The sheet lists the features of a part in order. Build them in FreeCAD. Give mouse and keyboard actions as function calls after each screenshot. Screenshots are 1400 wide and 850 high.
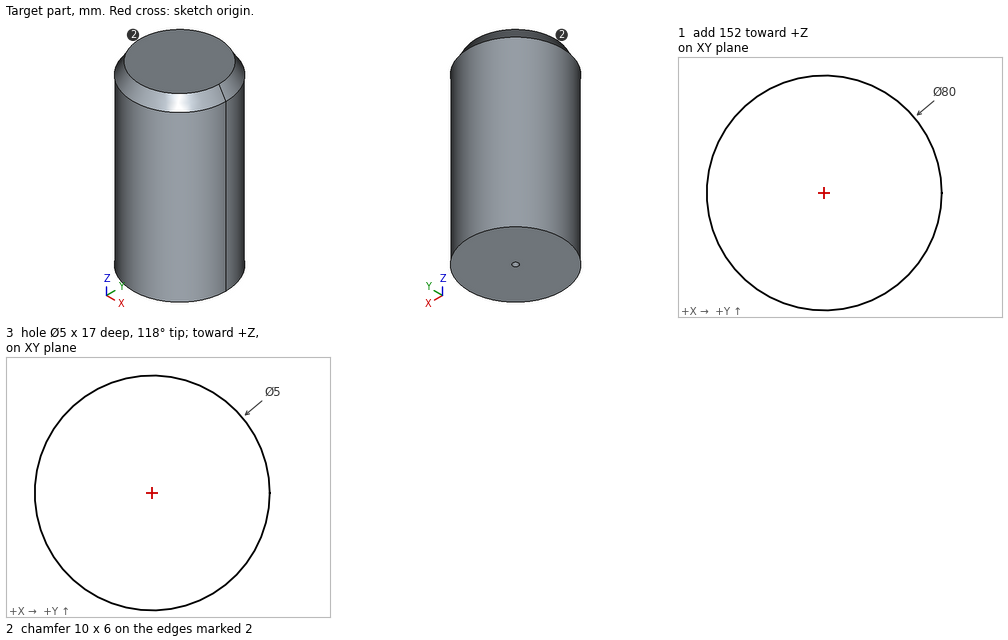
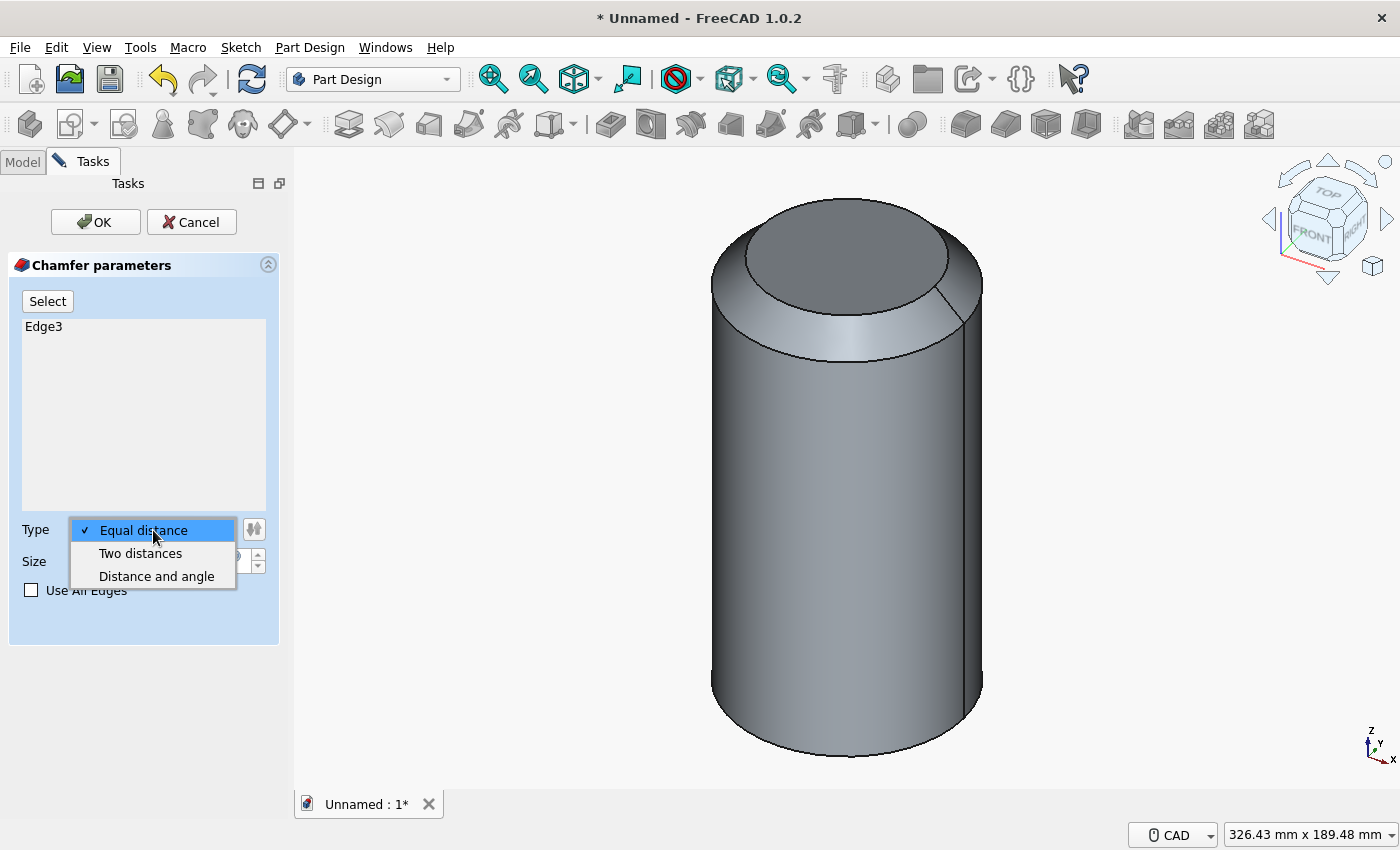
click(152, 554)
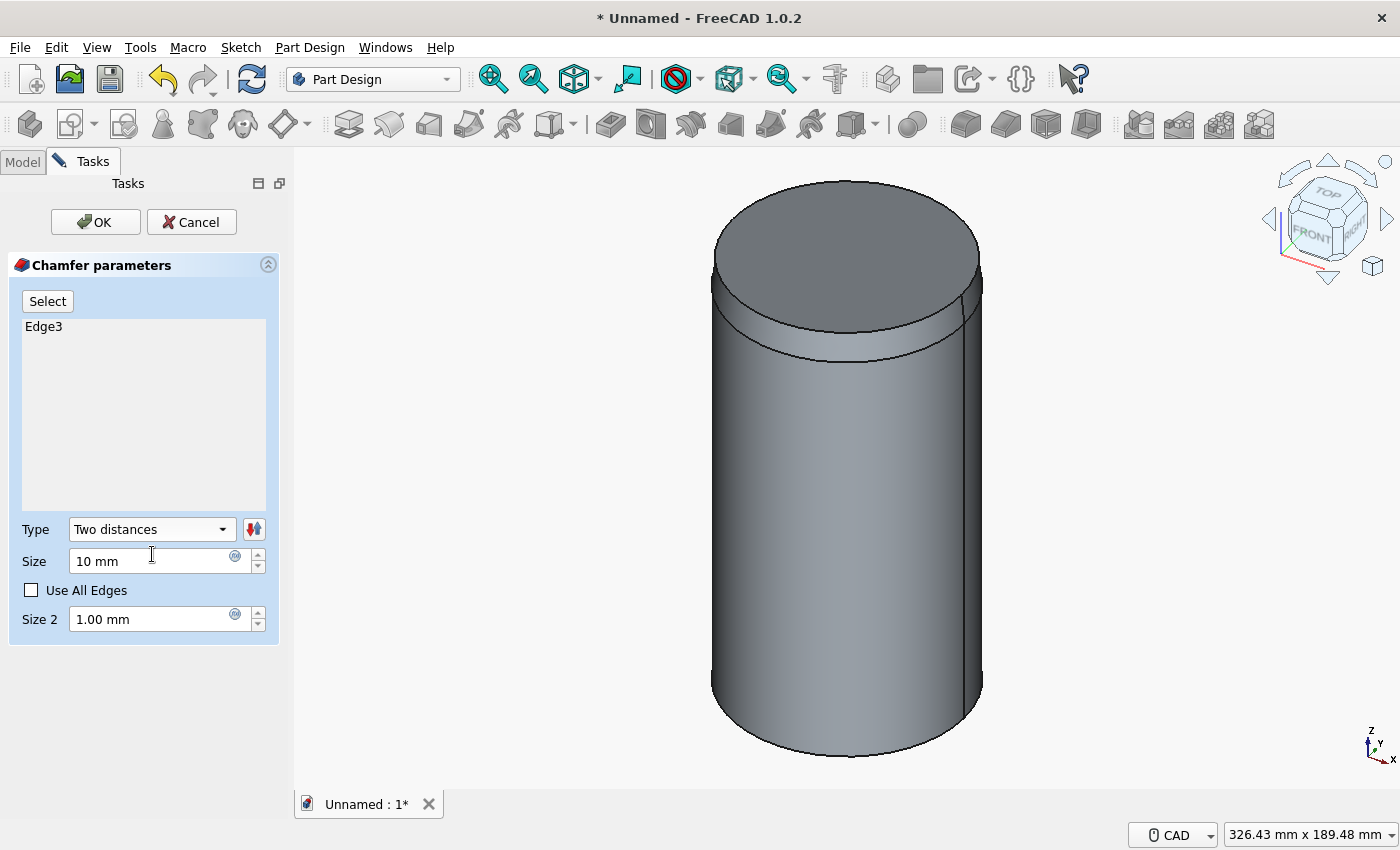
triple_click(160, 619)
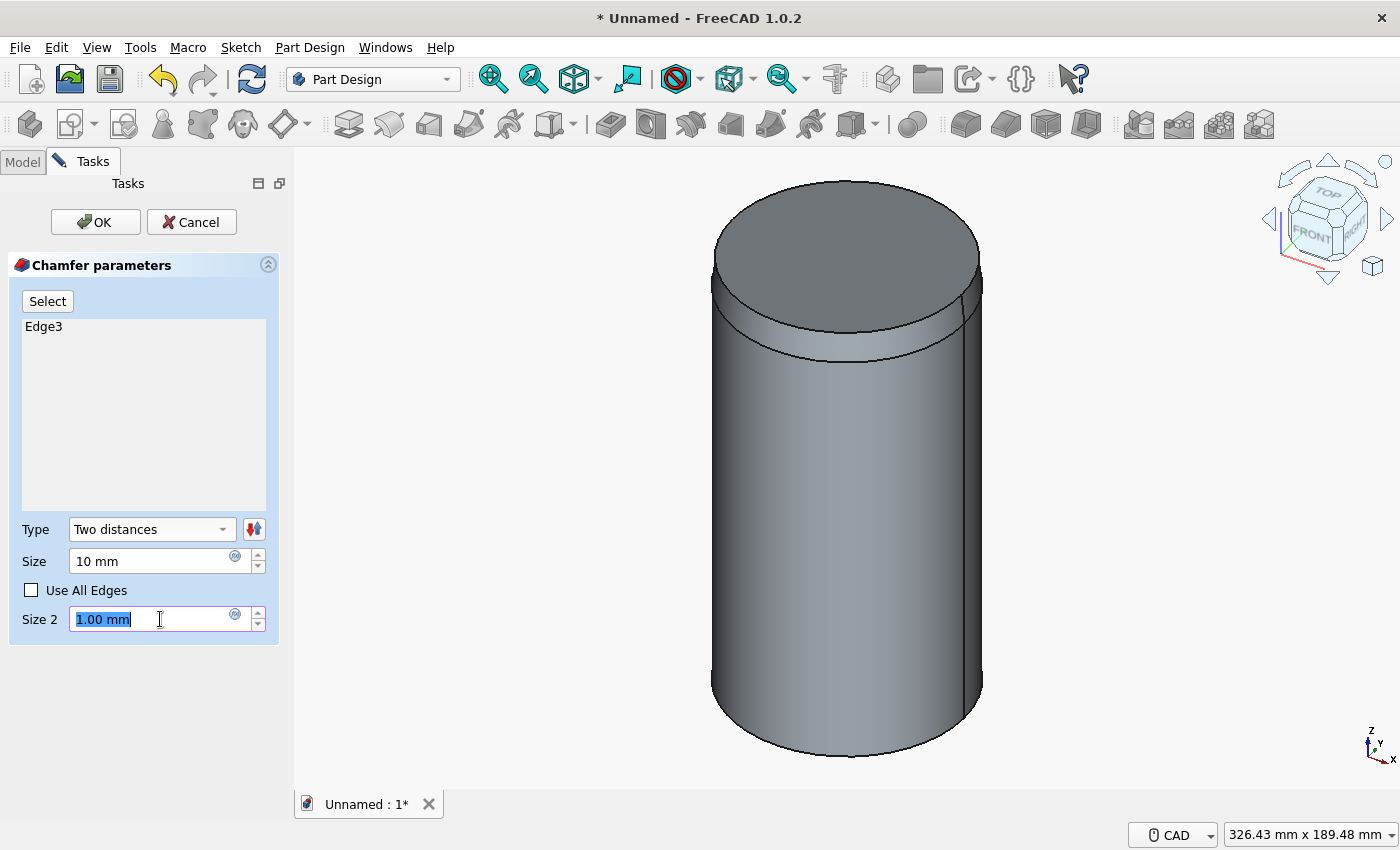
text(6)
key(Tab)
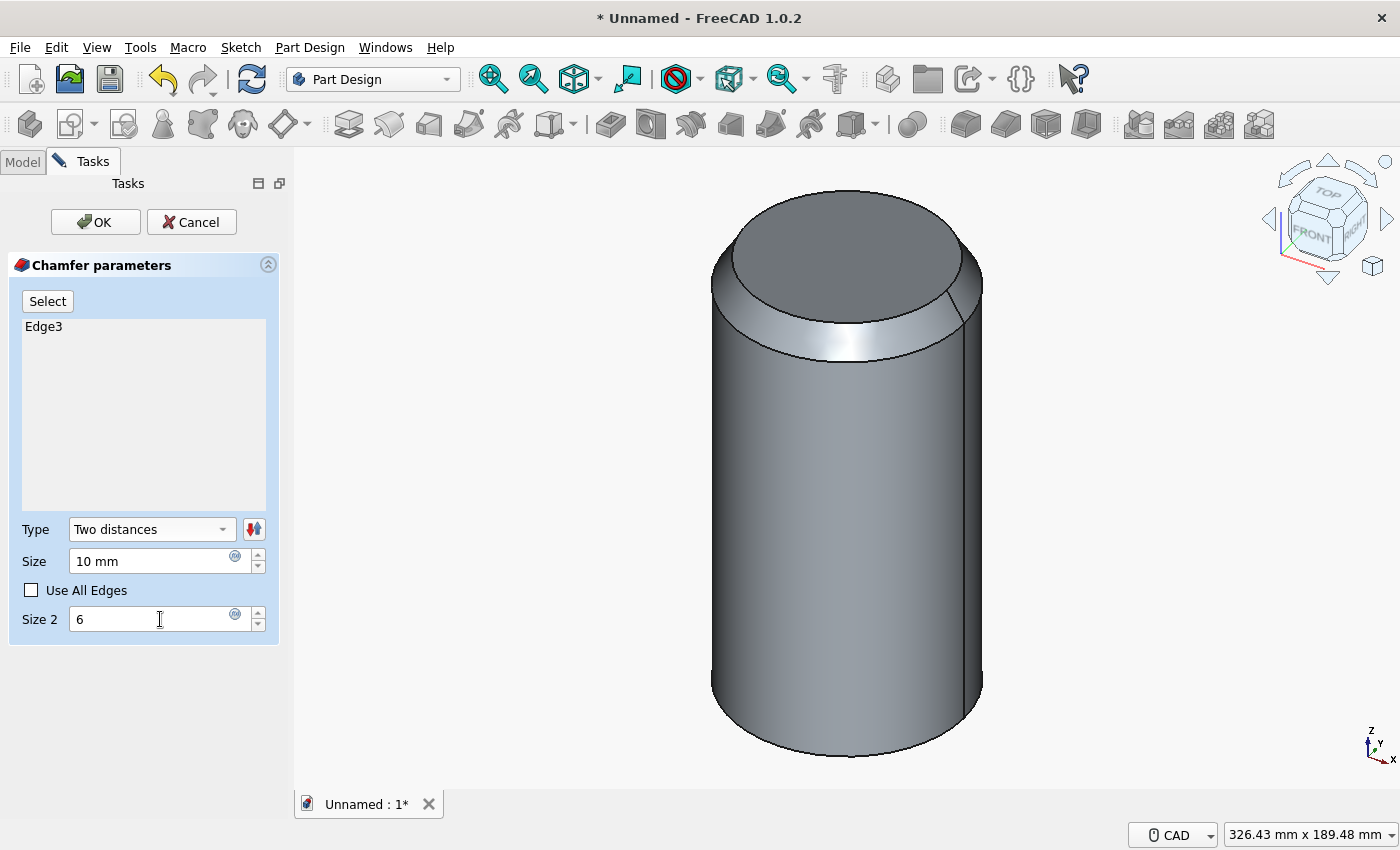
click(96, 222)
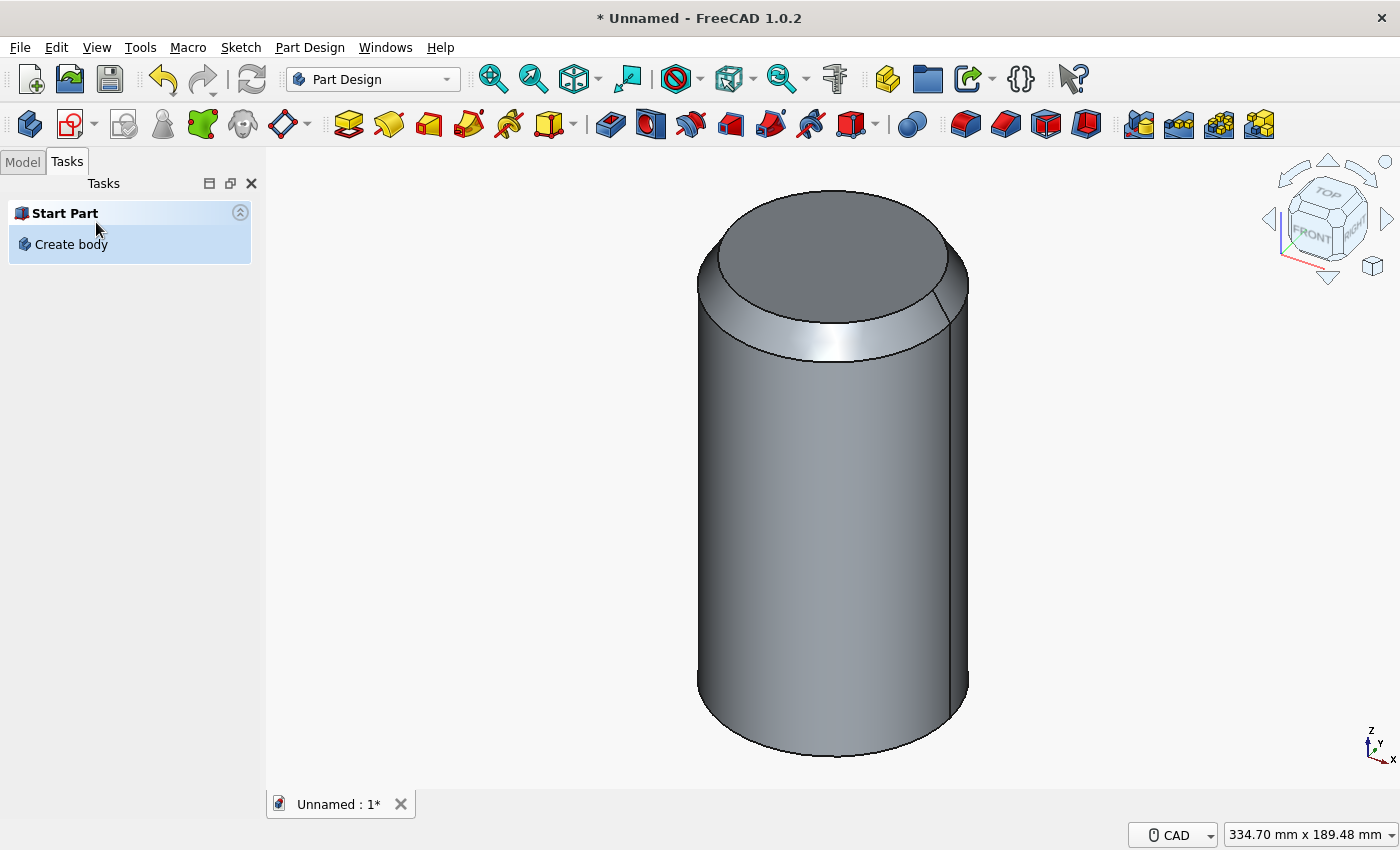
click(70, 124)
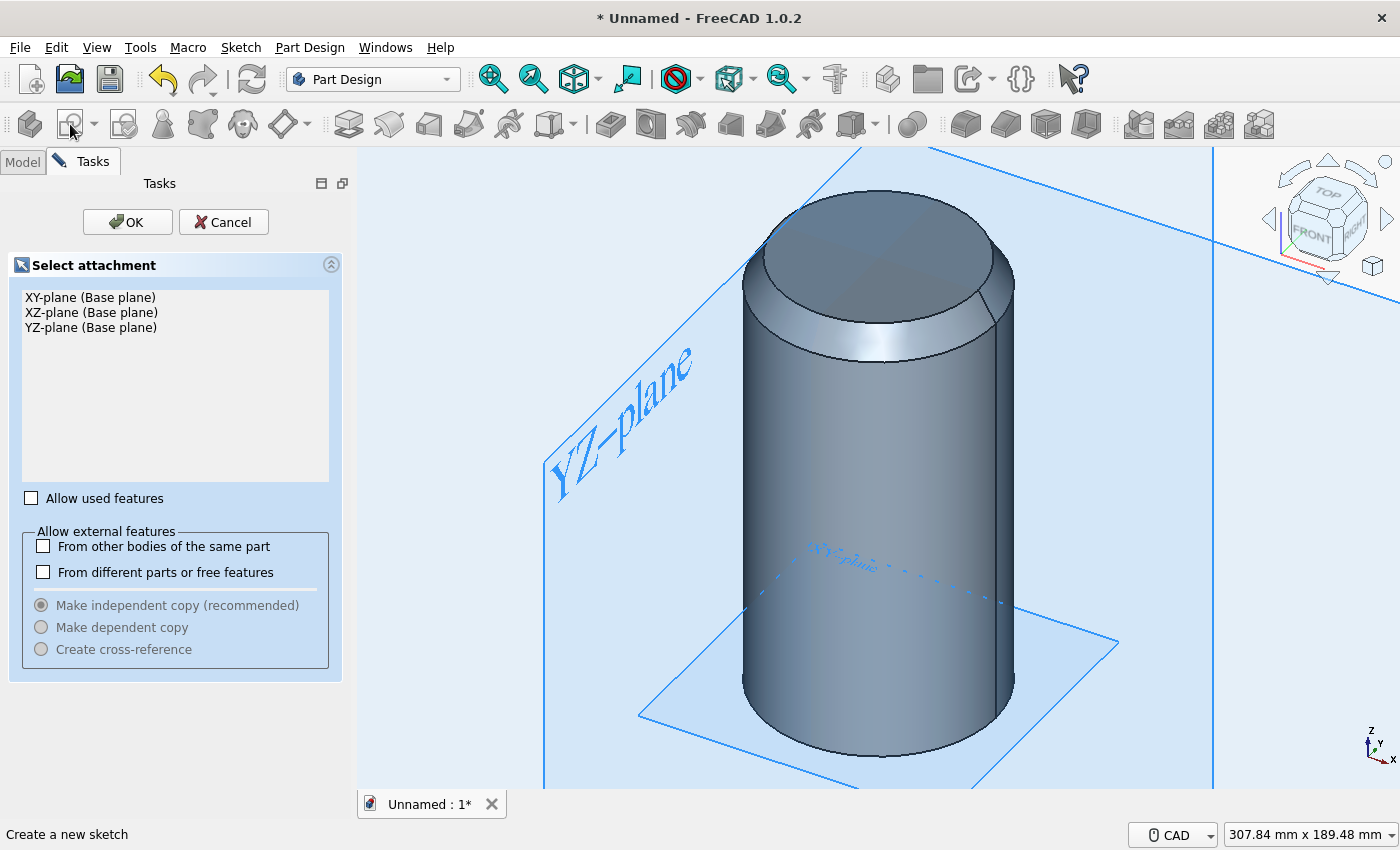
click(82, 298)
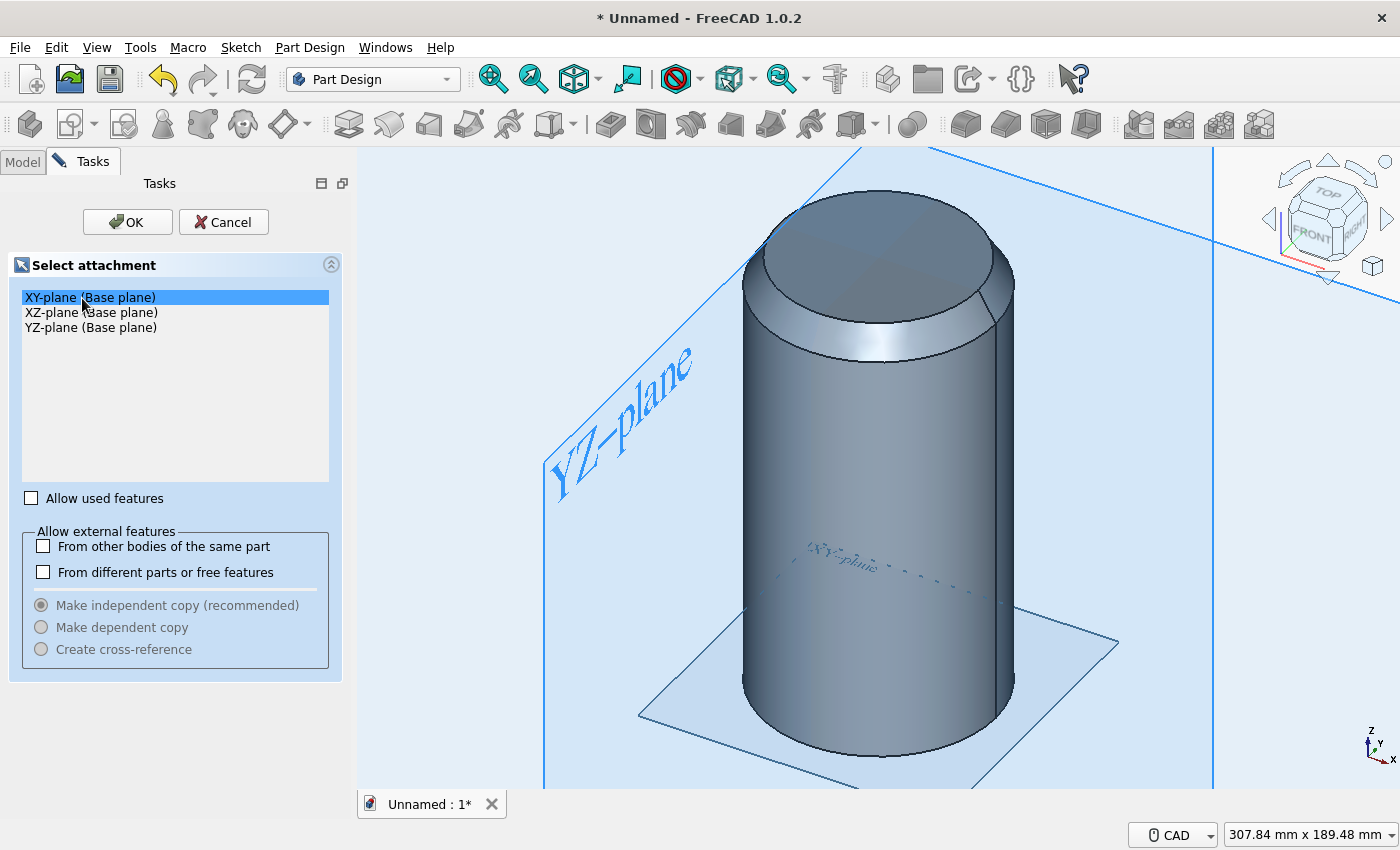
click(128, 222)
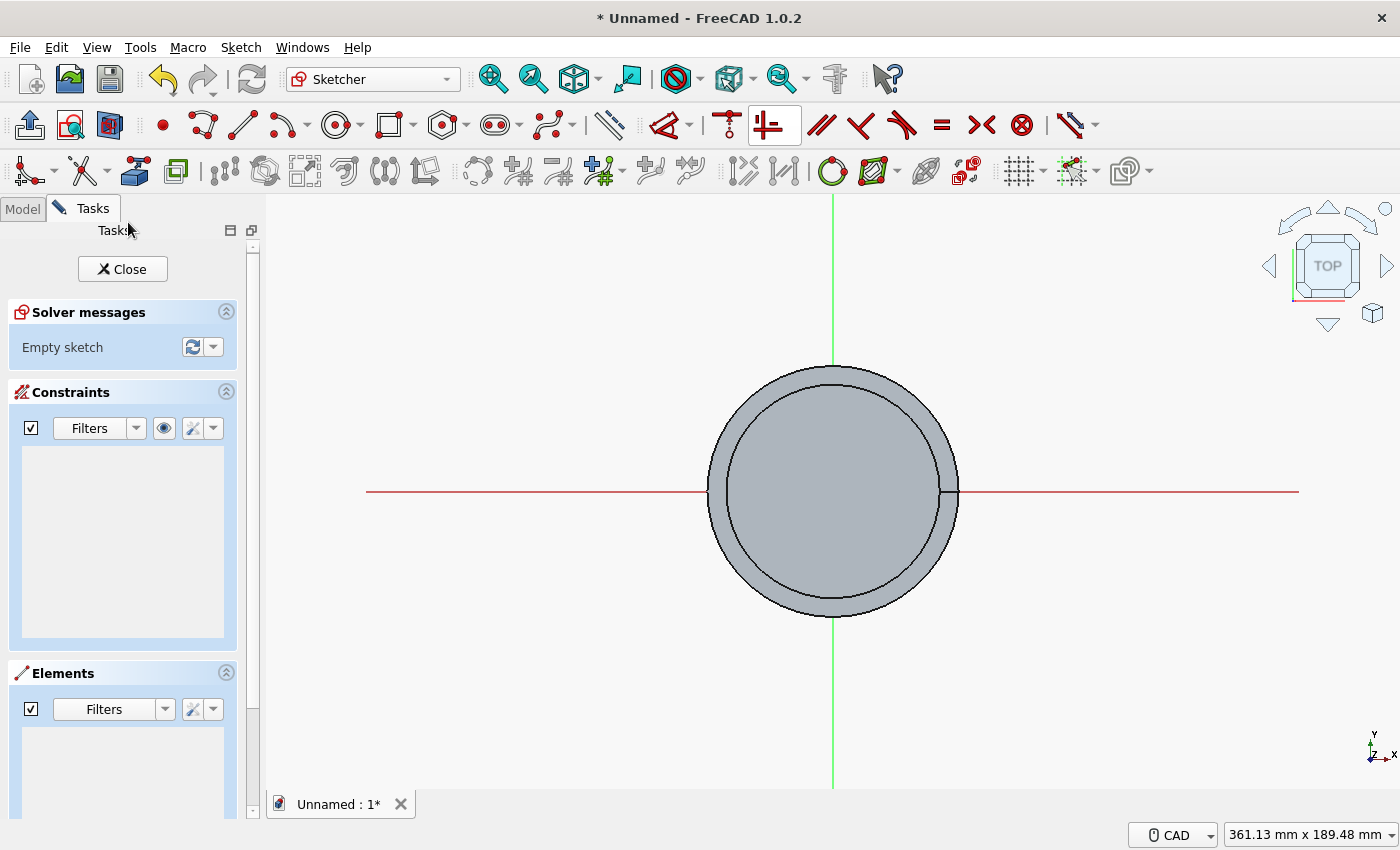
key(q)
key(s)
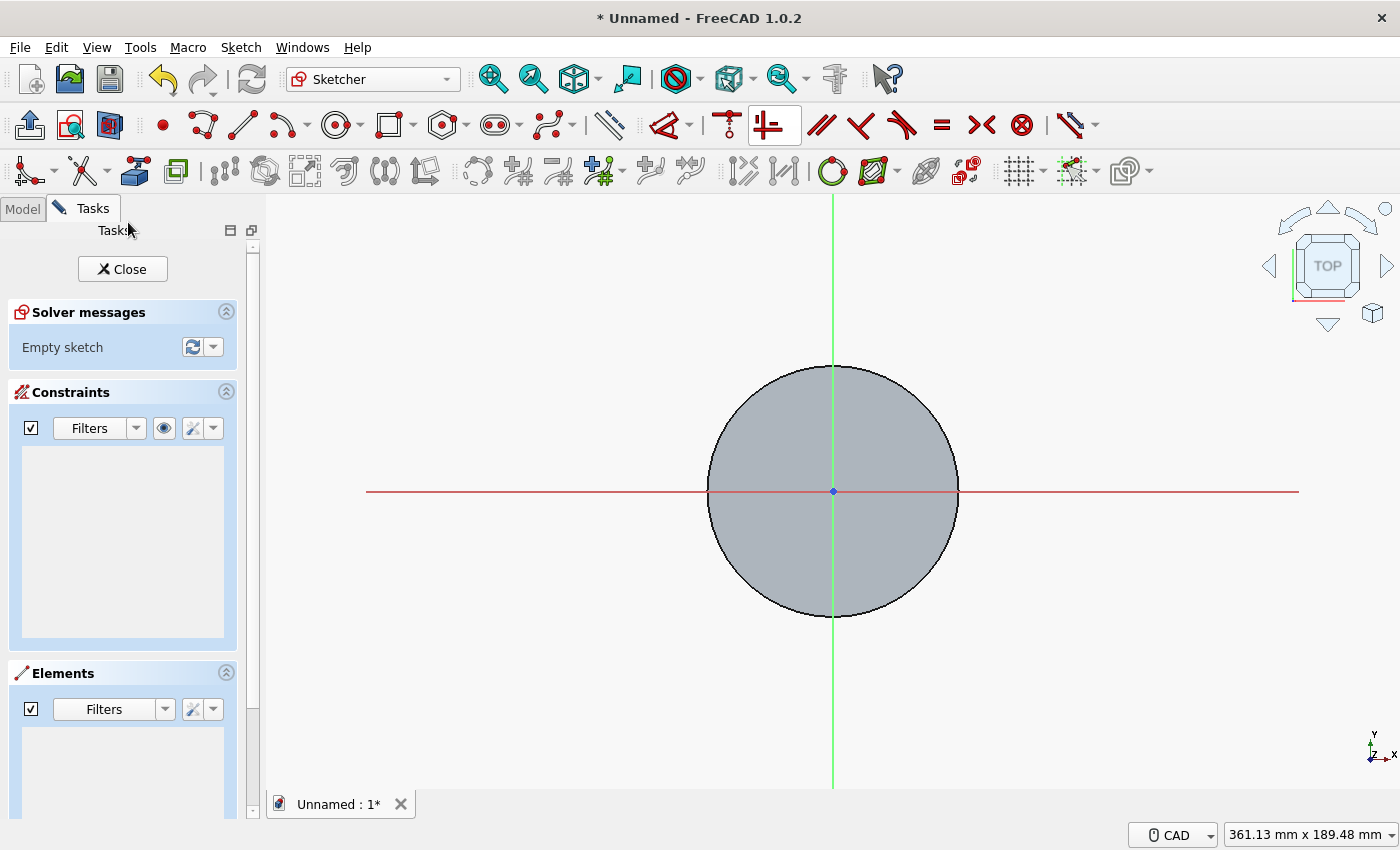
scroll(837, 492, up, 15)